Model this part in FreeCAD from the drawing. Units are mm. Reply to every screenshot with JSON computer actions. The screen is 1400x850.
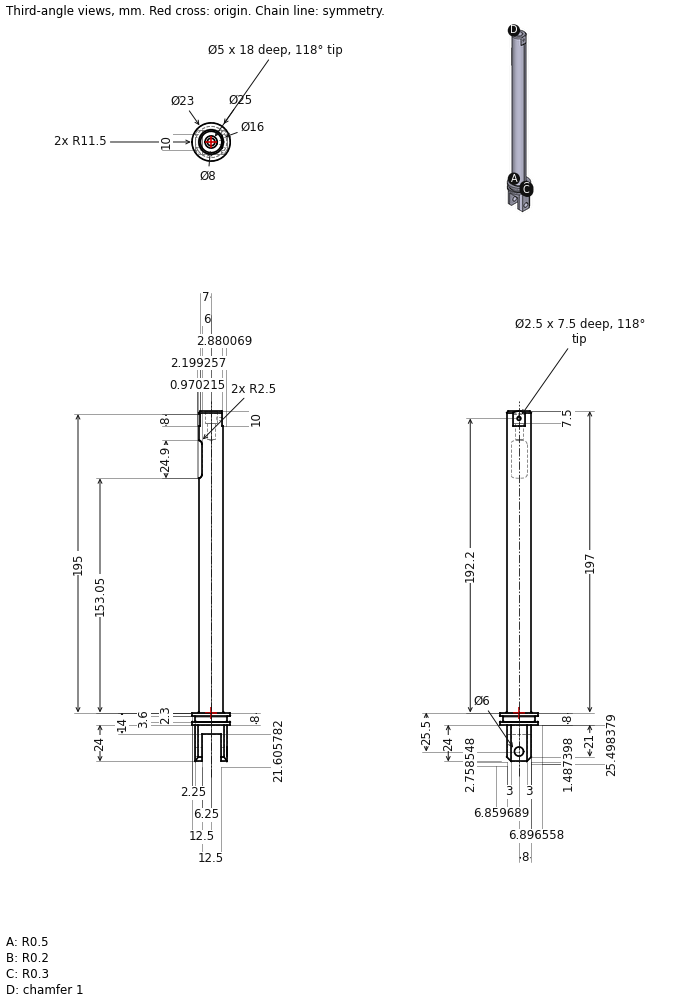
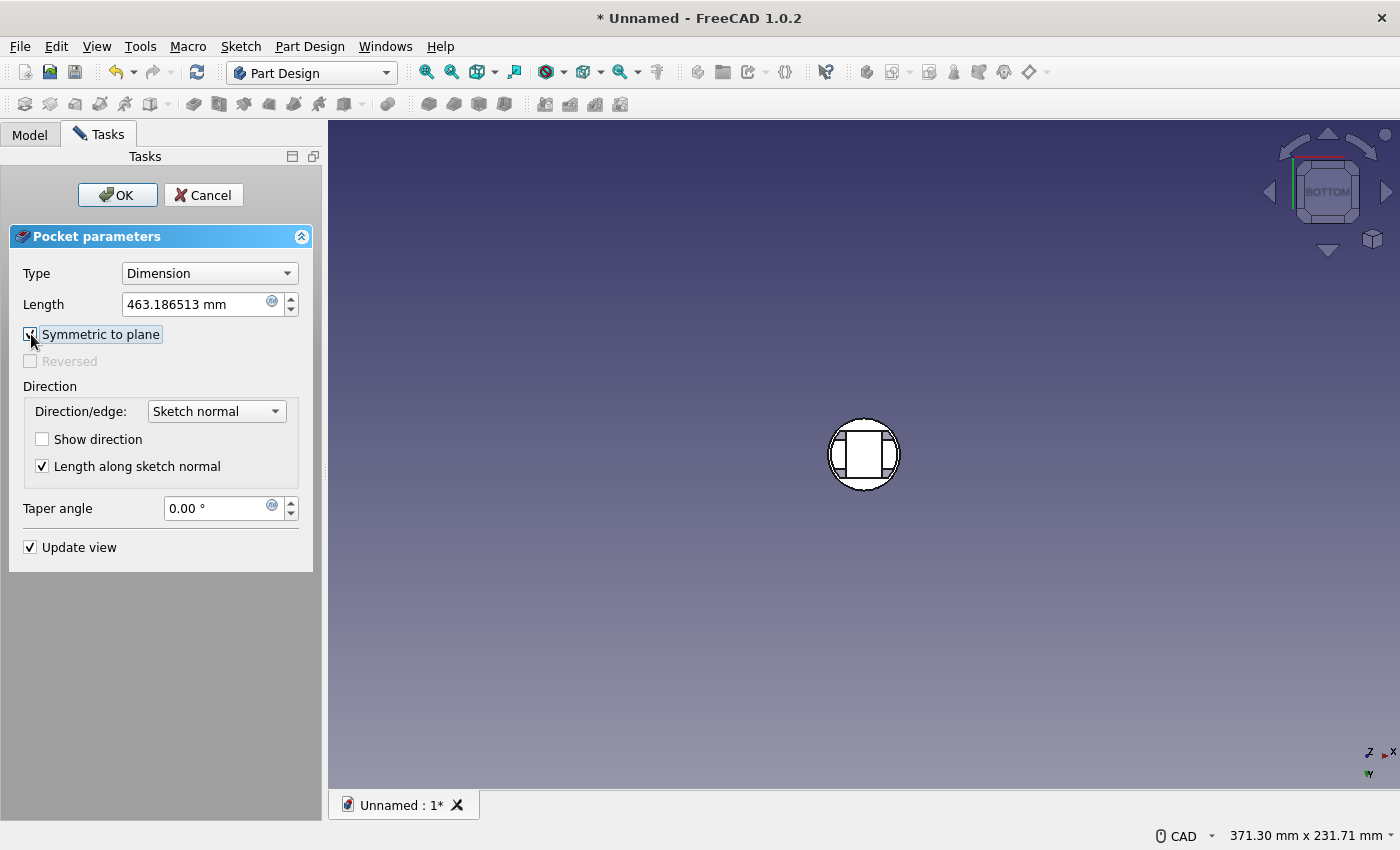
{"action": "left_click", "coordinate": [118, 195]}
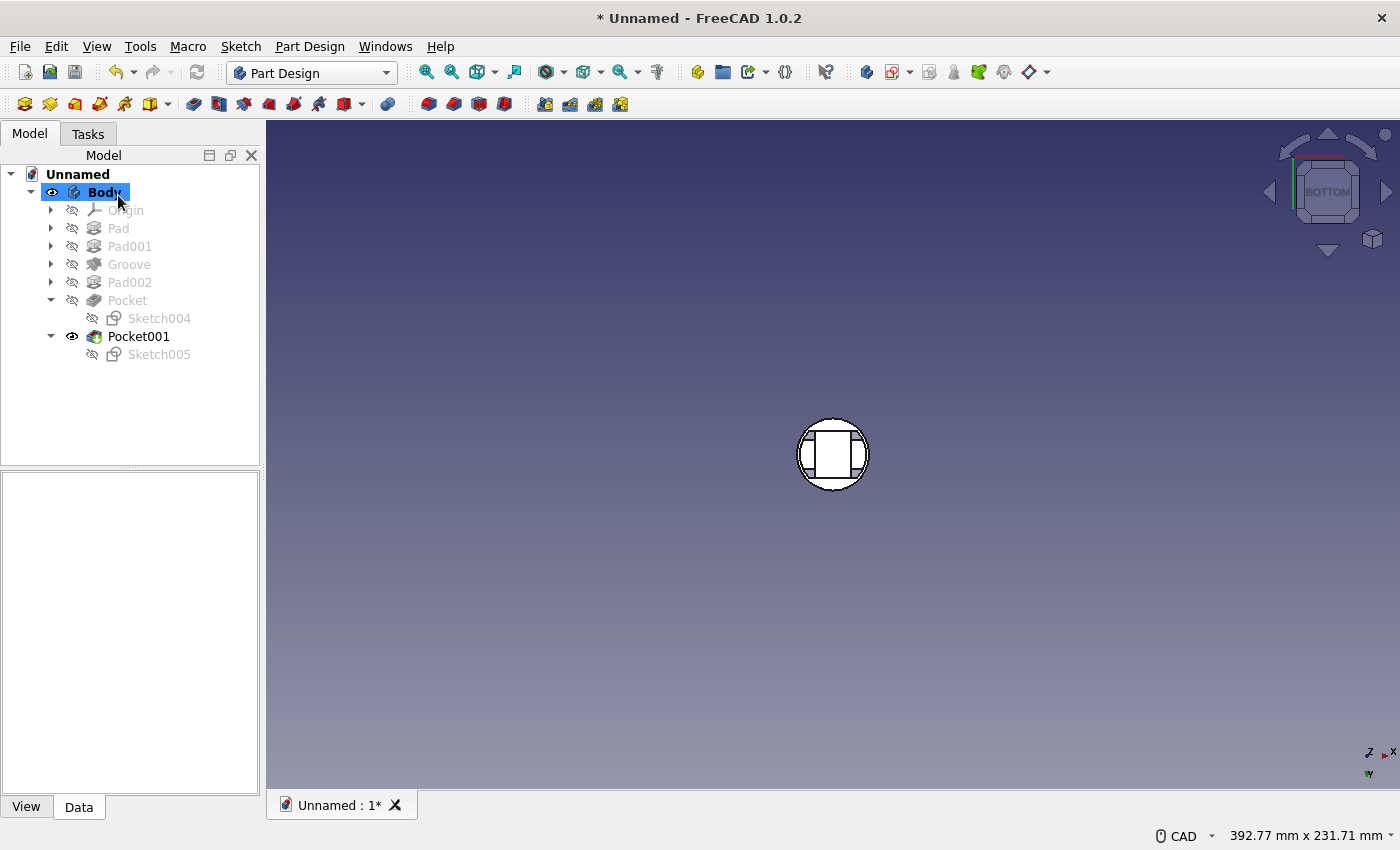
{"action": "left_click", "coordinate": [427, 72]}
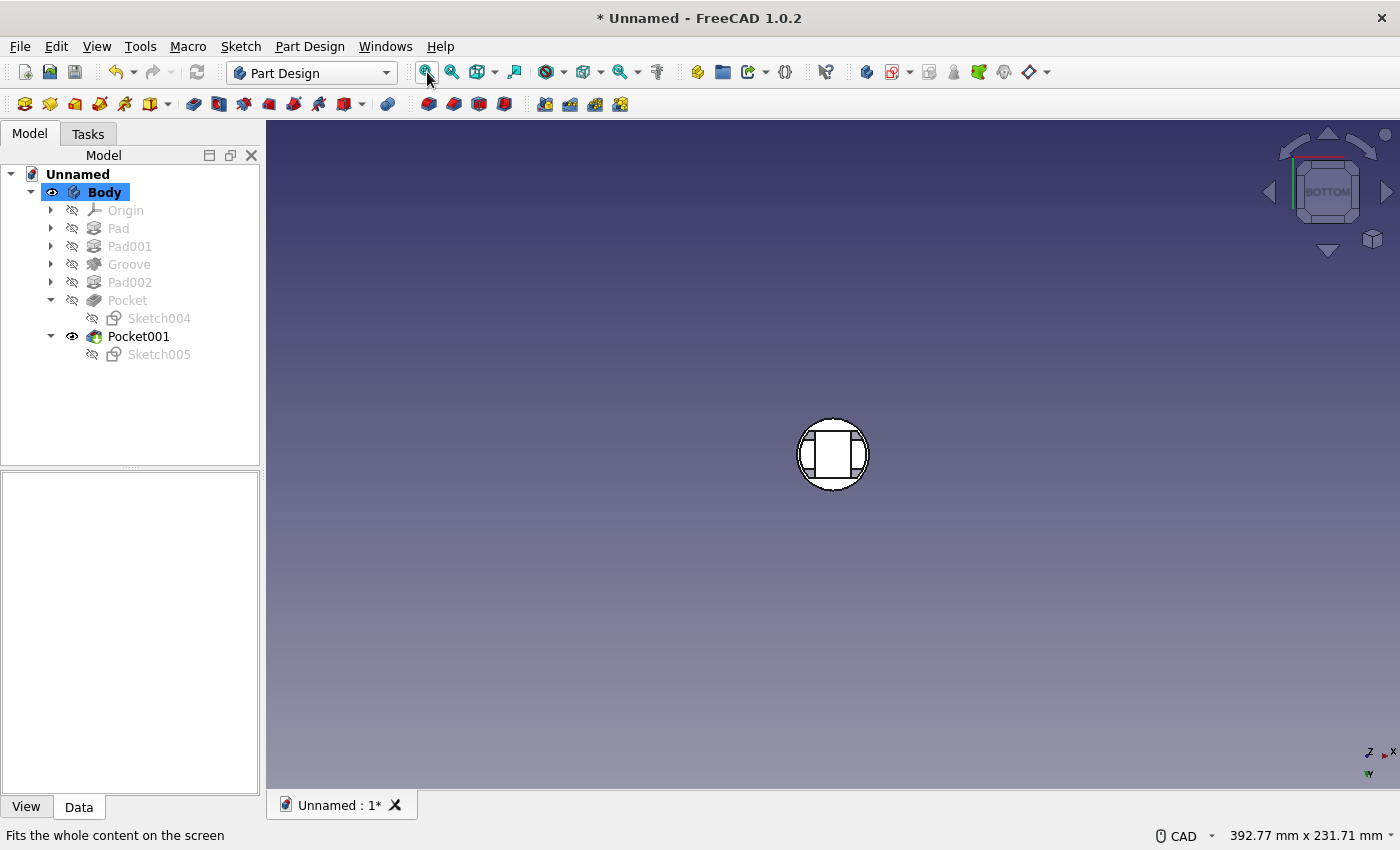
{"action": "scroll", "coordinate": [833, 423], "scroll_direction": "up", "scroll_amount": 5}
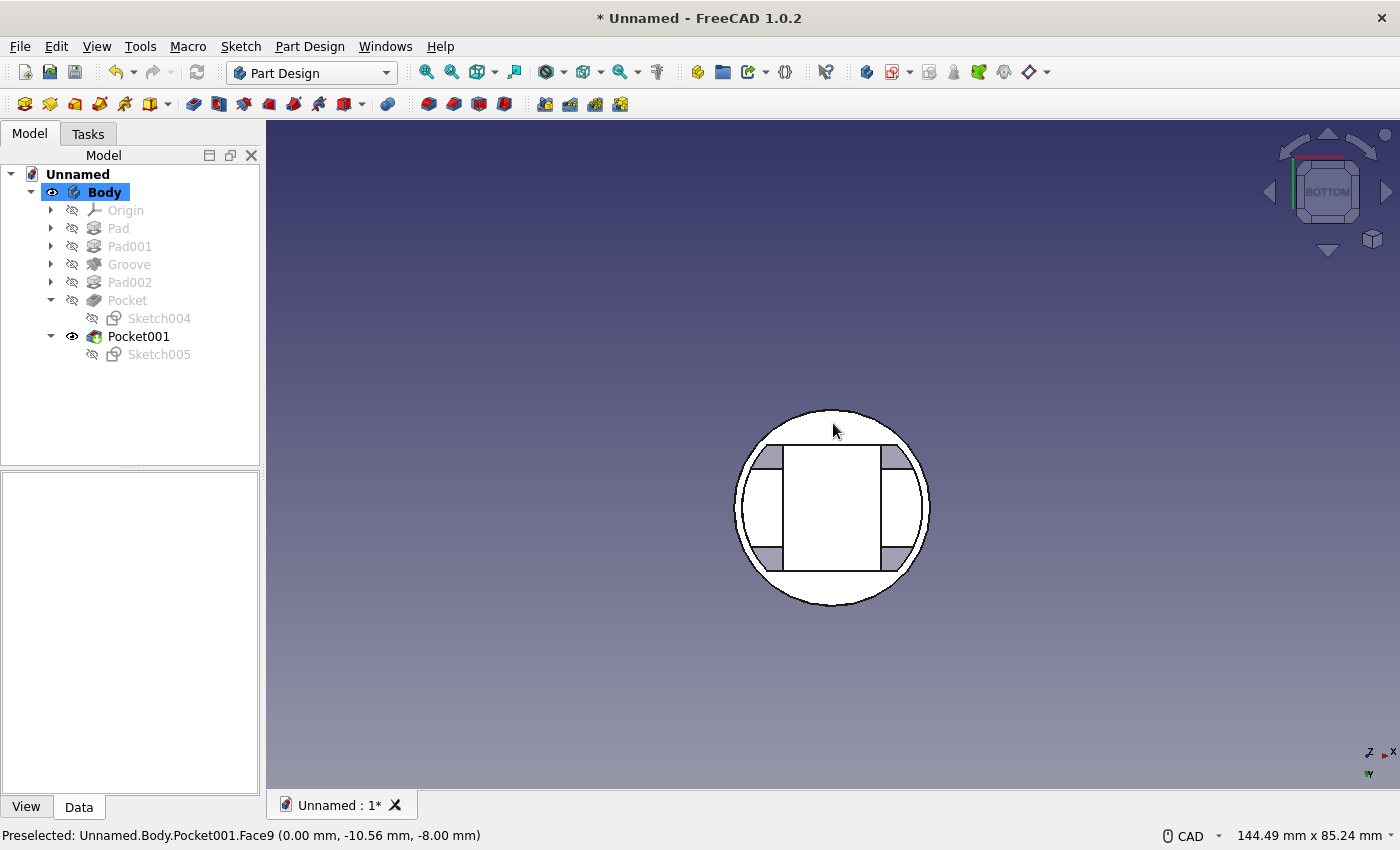
{"action": "left_click", "coordinate": [832, 423]}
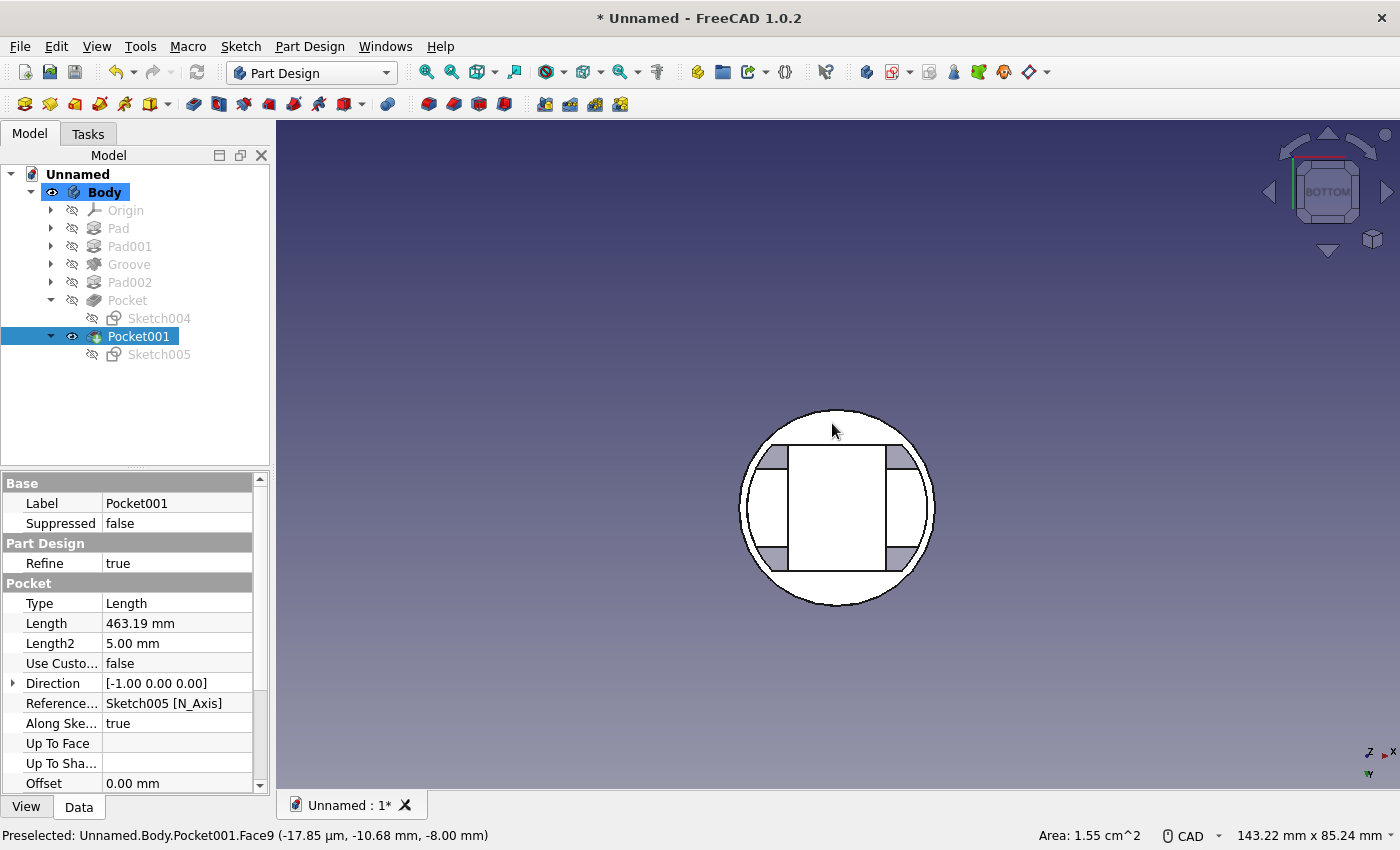
{"action": "left_click", "coordinate": [892, 72]}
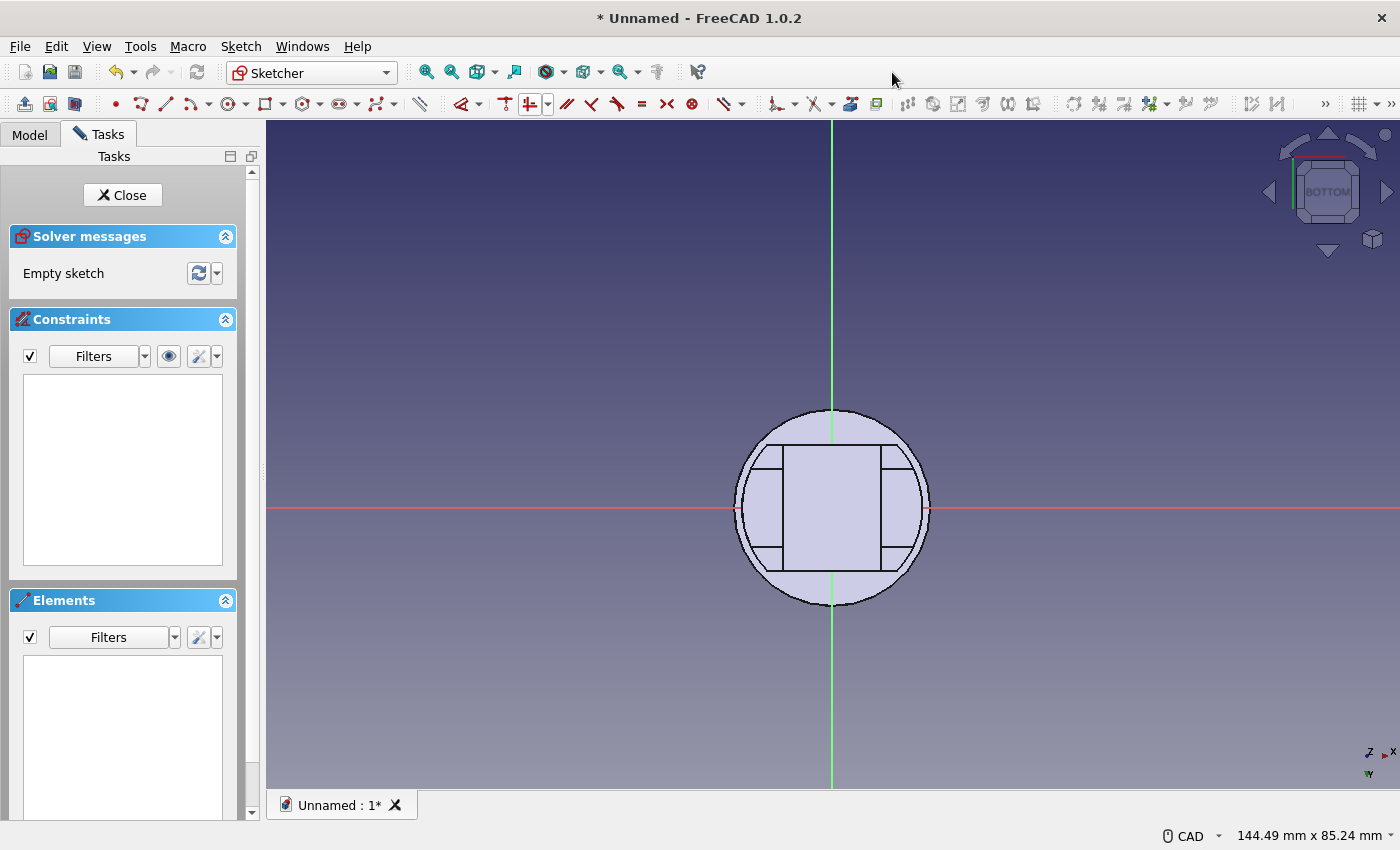
{"action": "left_click", "coordinate": [75, 104]}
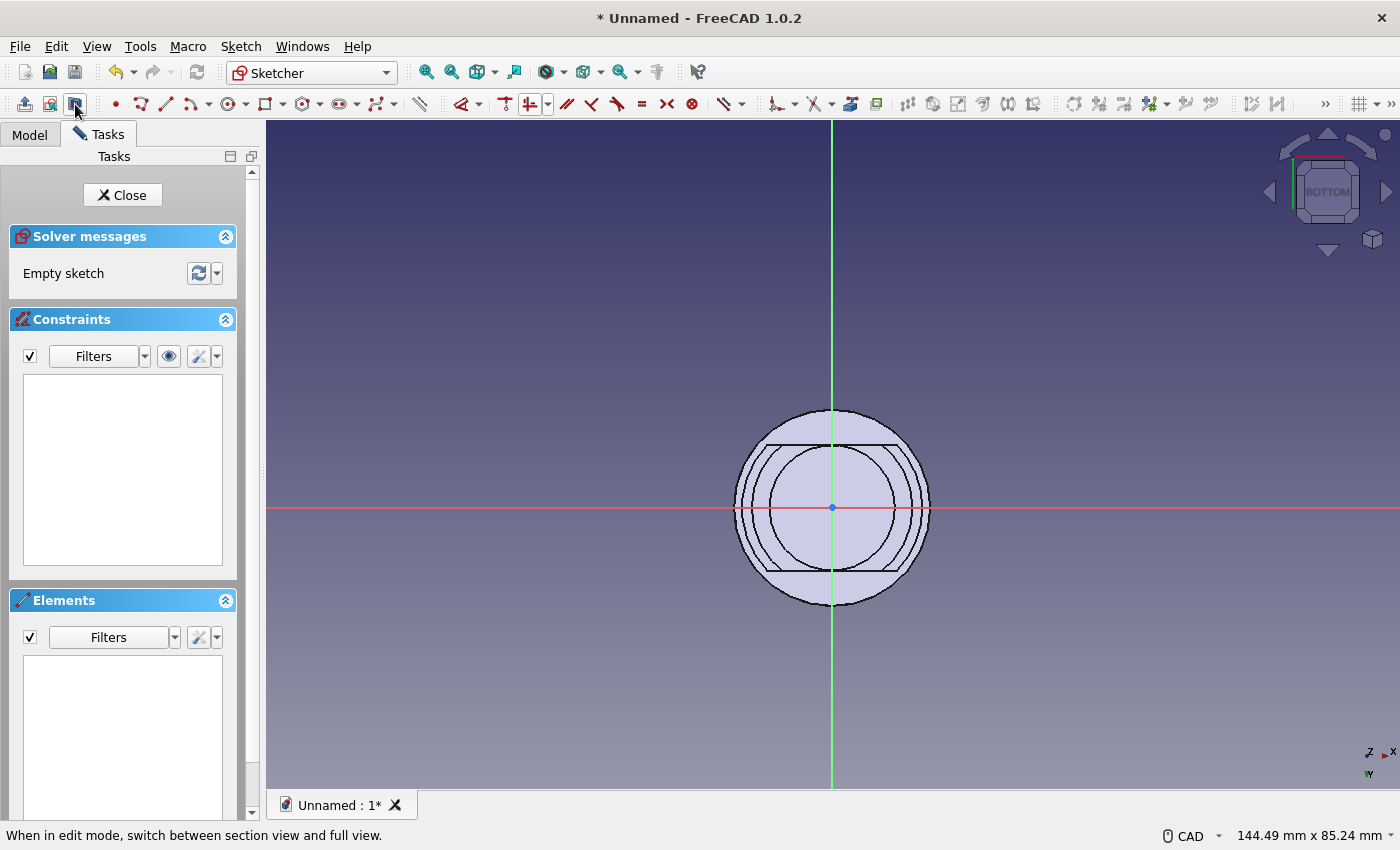
{"action": "scroll", "coordinate": [854, 525], "scroll_direction": "up", "scroll_amount": 7}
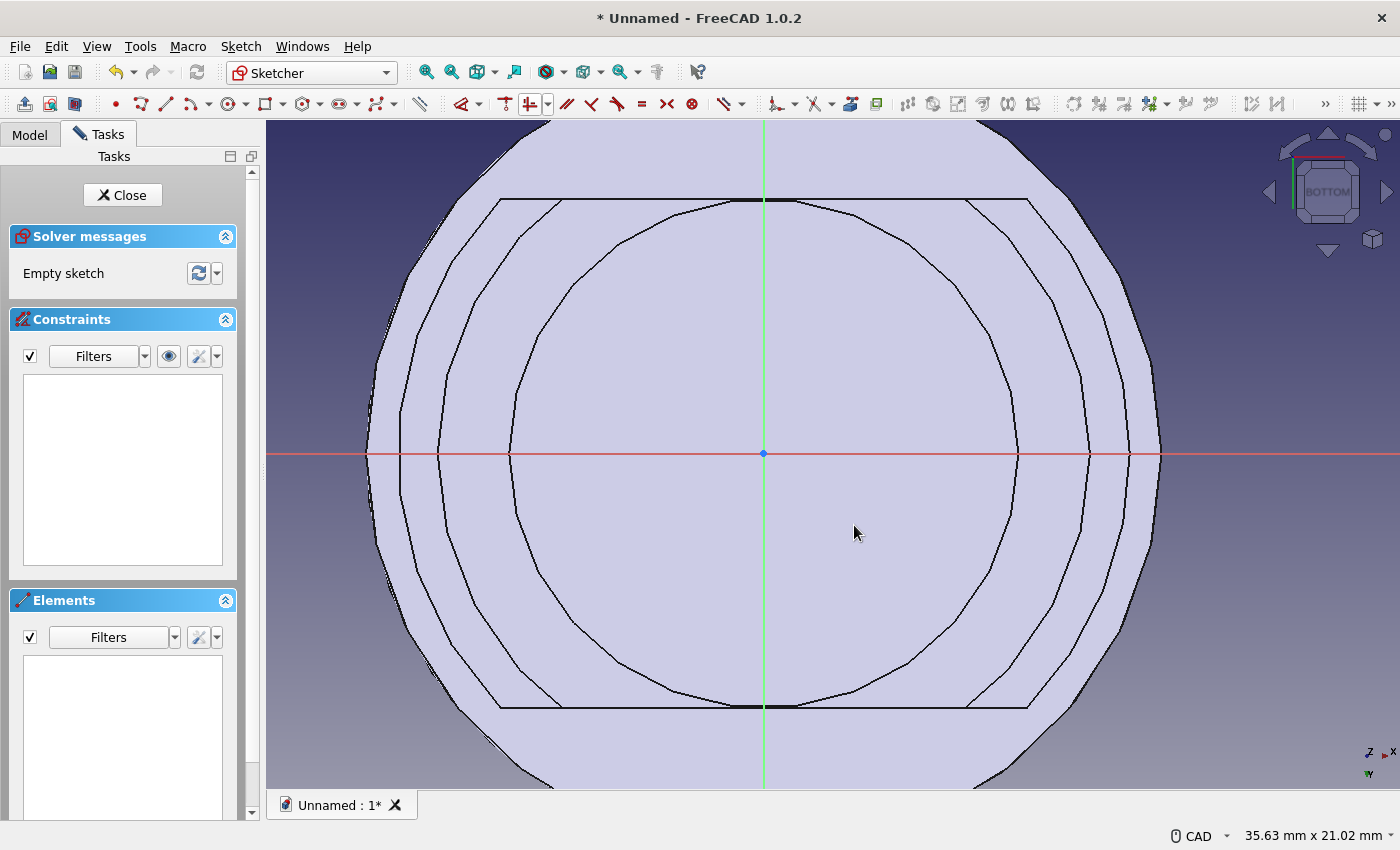
{"action": "left_click", "coordinate": [166, 104]}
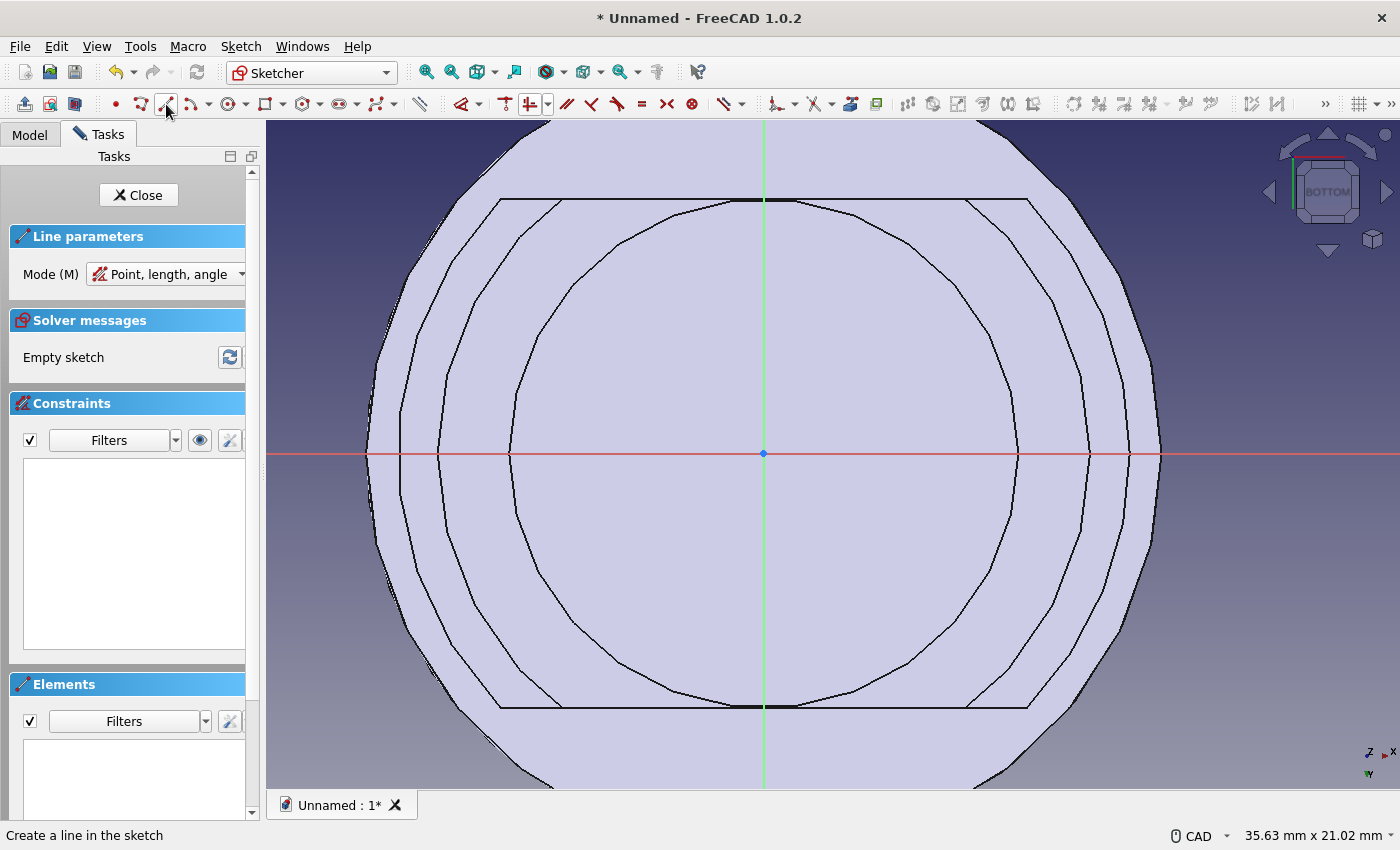
{"action": "left_click", "coordinate": [434, 613]}
{"action": "left_click", "coordinate": [434, 294]}